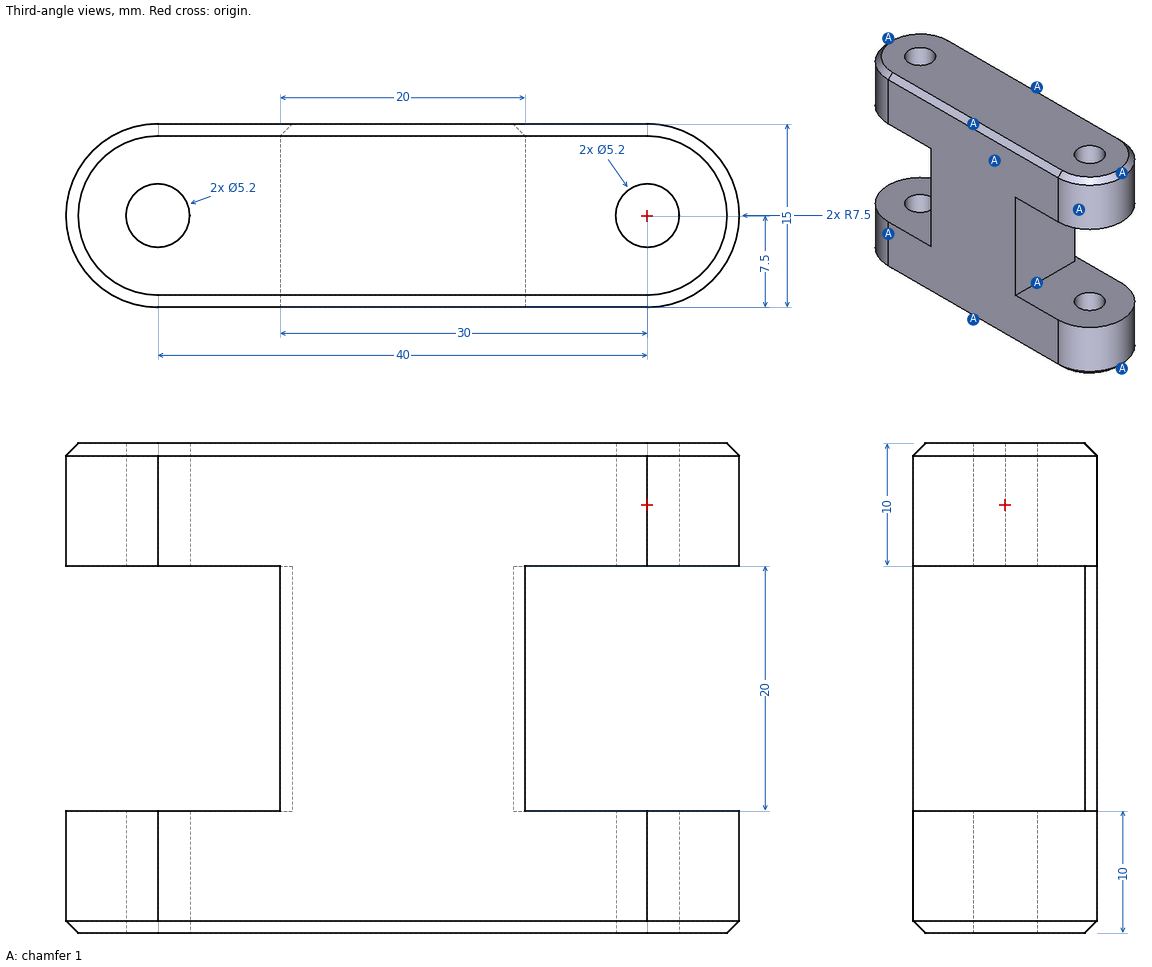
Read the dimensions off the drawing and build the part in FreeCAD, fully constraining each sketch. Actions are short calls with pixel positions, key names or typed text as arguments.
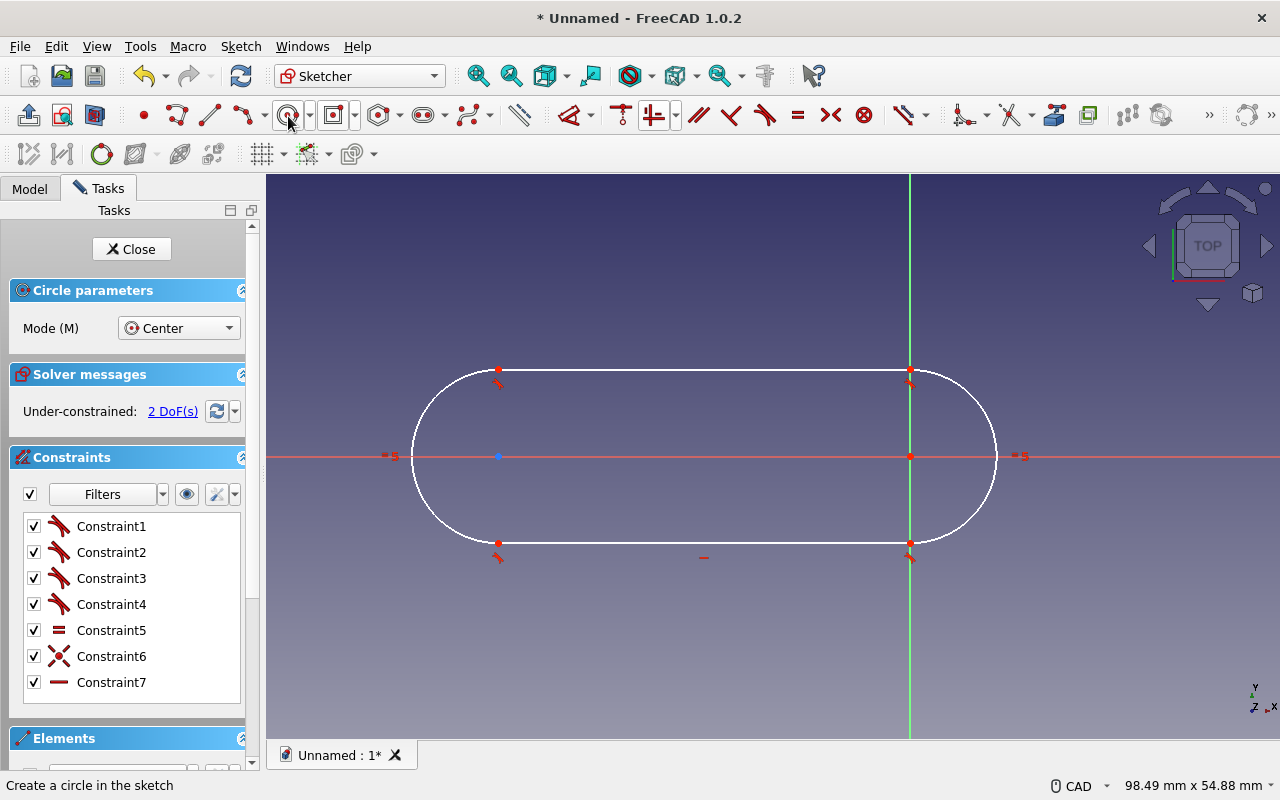
click(910, 456)
move(929, 438)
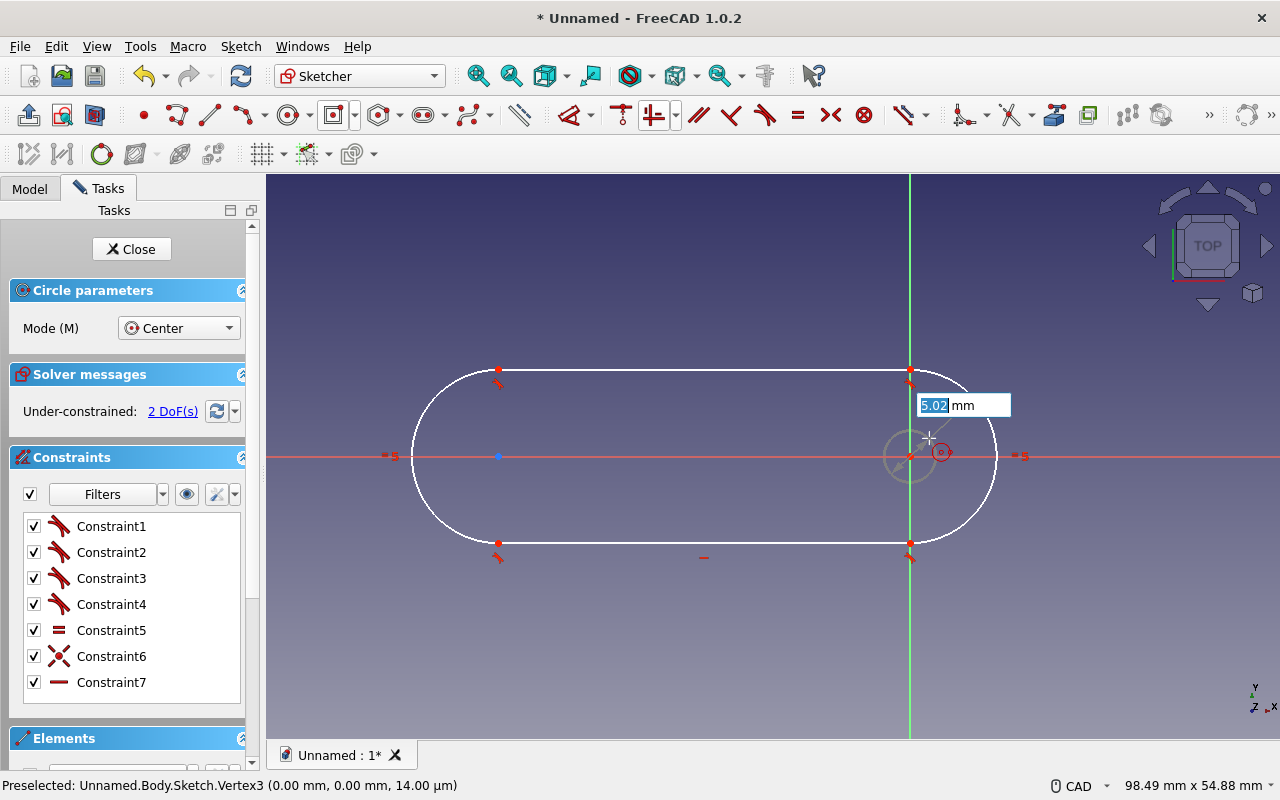
text(5.2)
key(Return)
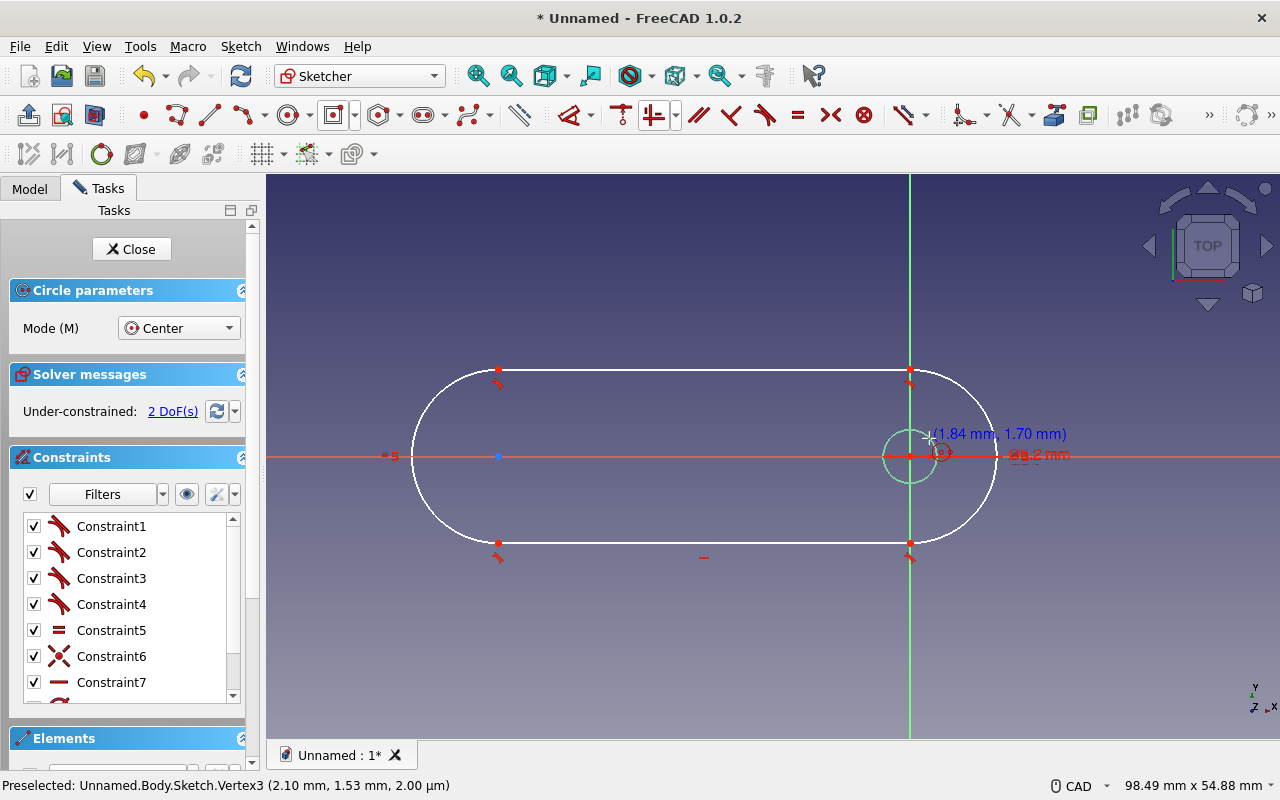
click(499, 456)
move(517, 438)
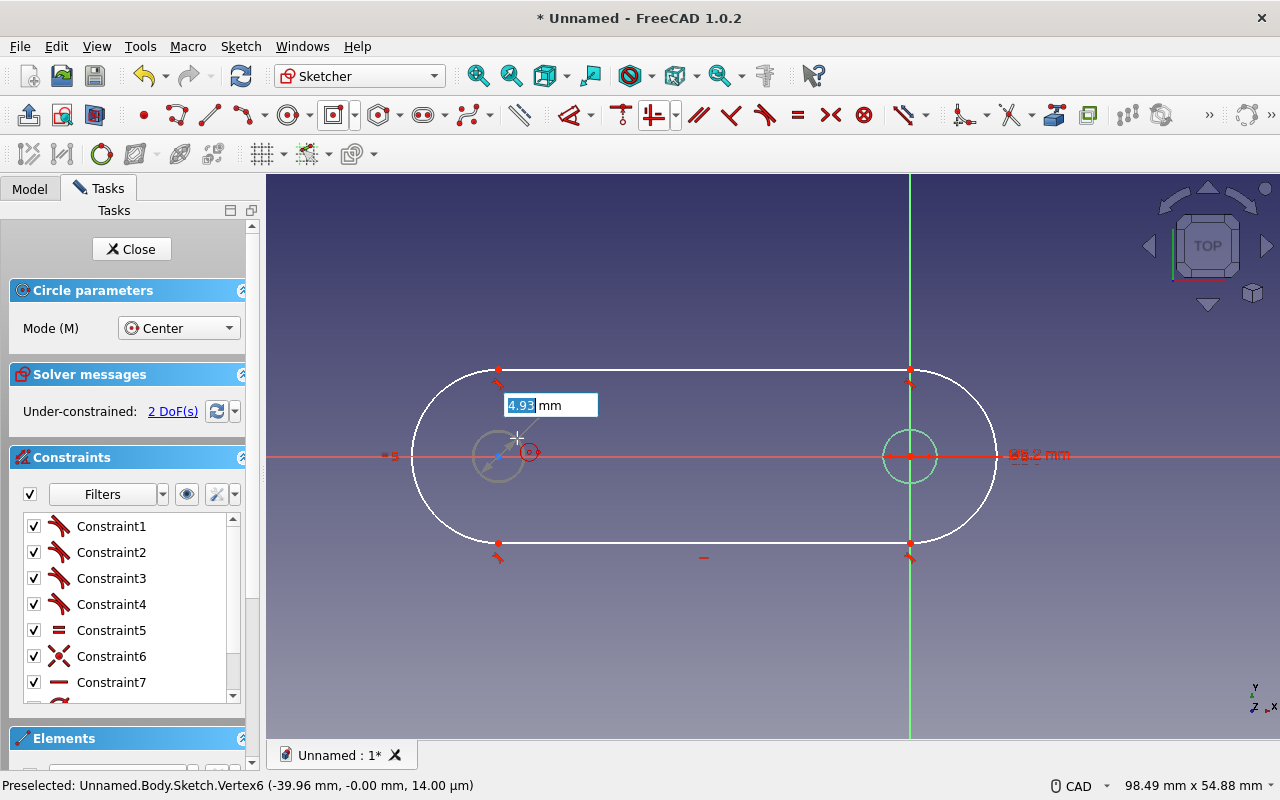
text(5.2)
key(Return)
key(Escape)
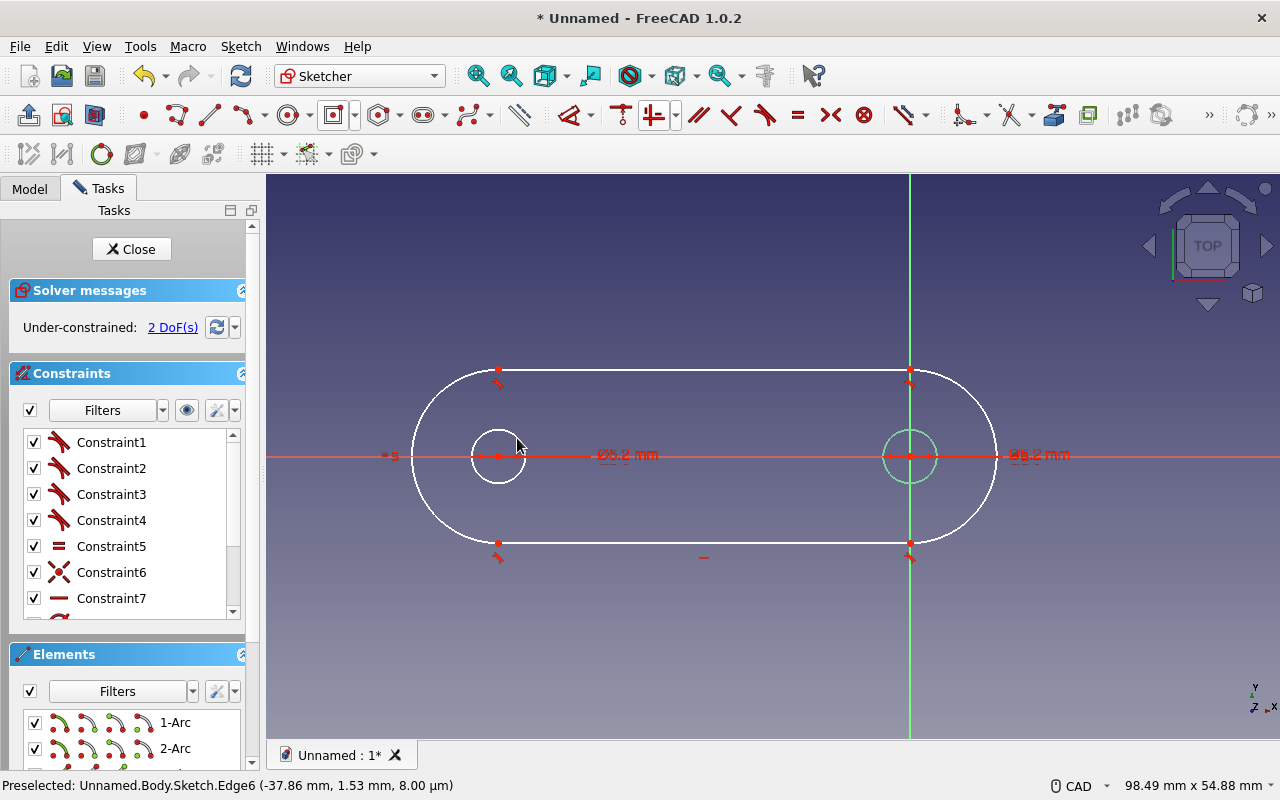
click(568, 116)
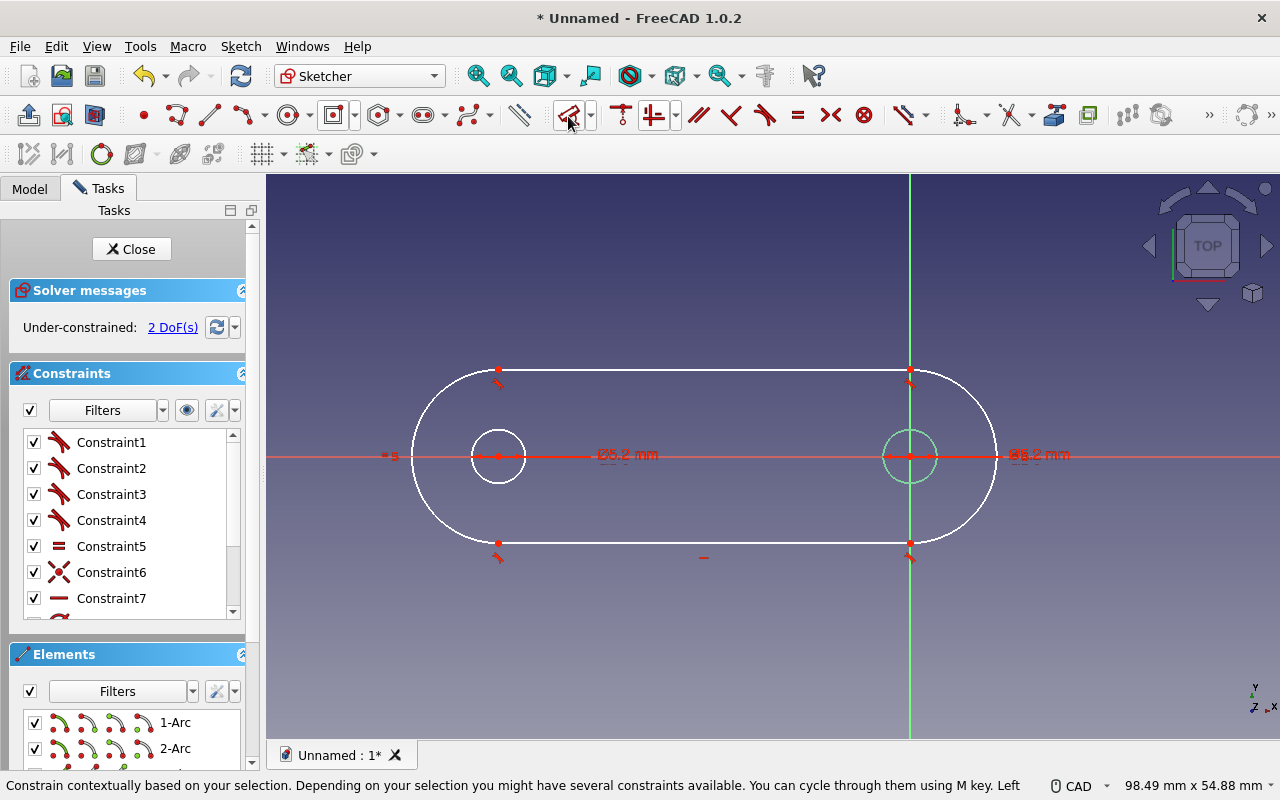
click(980, 507)
click(1006, 526)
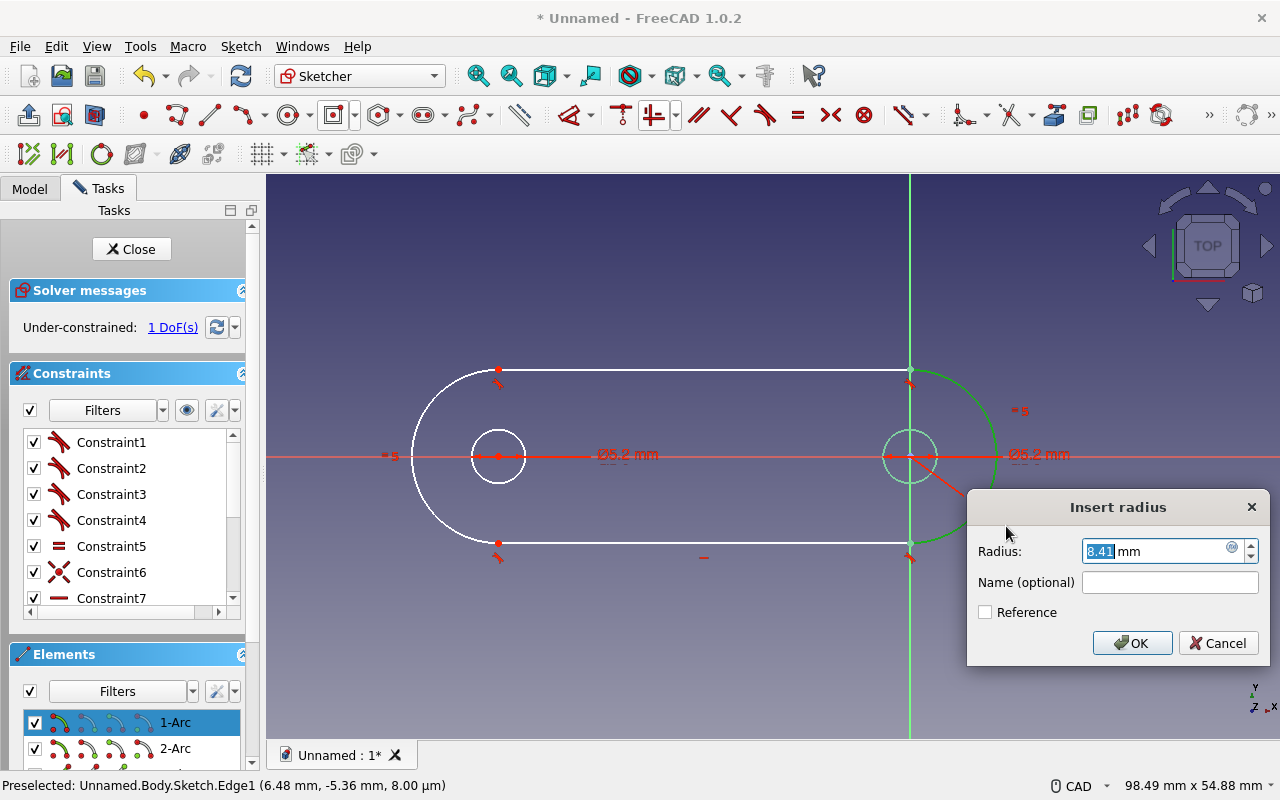
text(7.5)
key(Return)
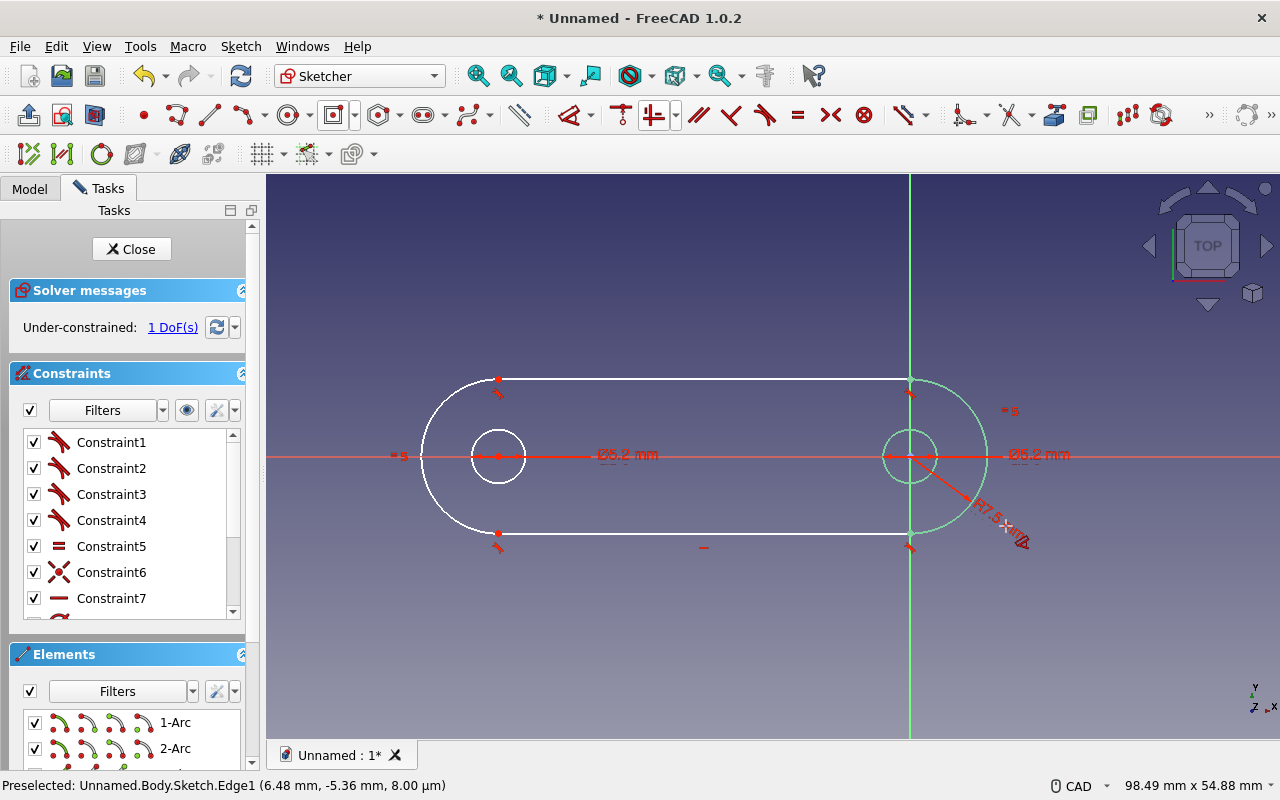
click(787, 534)
click(704, 568)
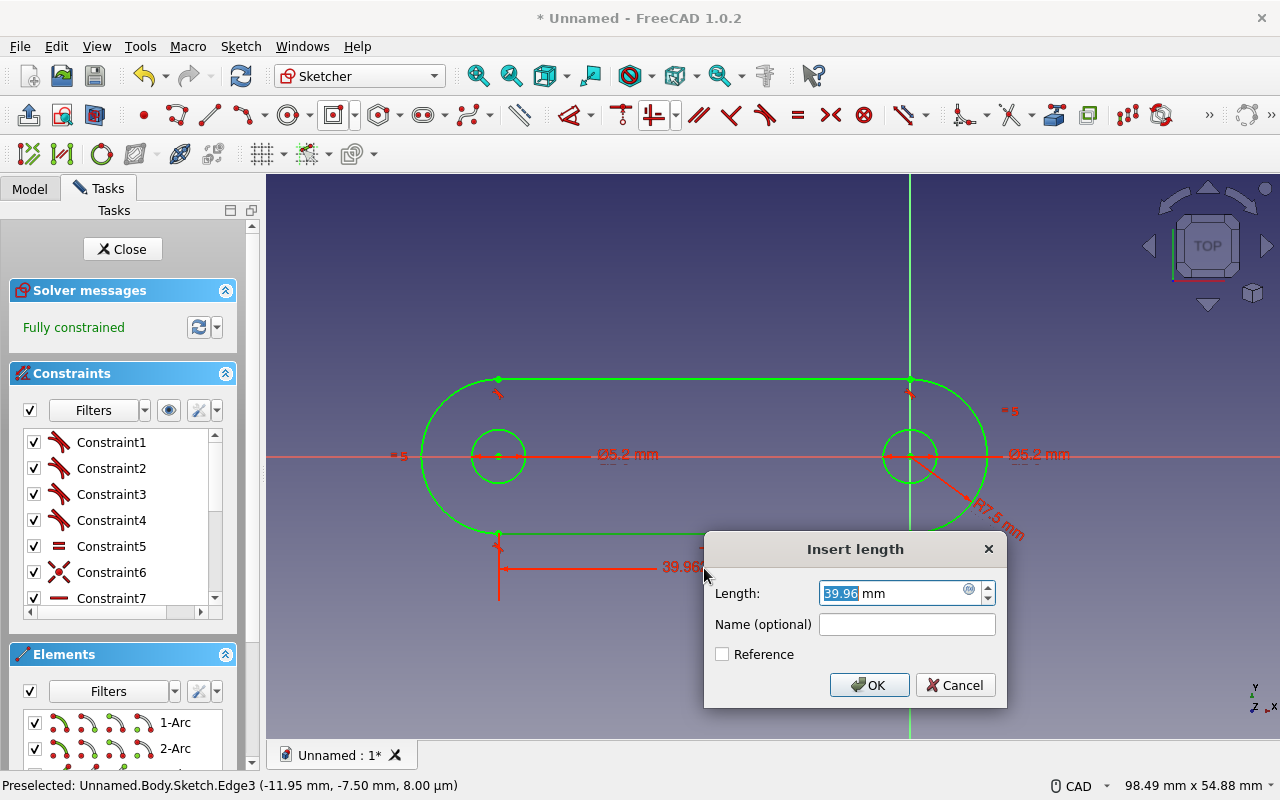
text(40)
key(Return)
key(Escape)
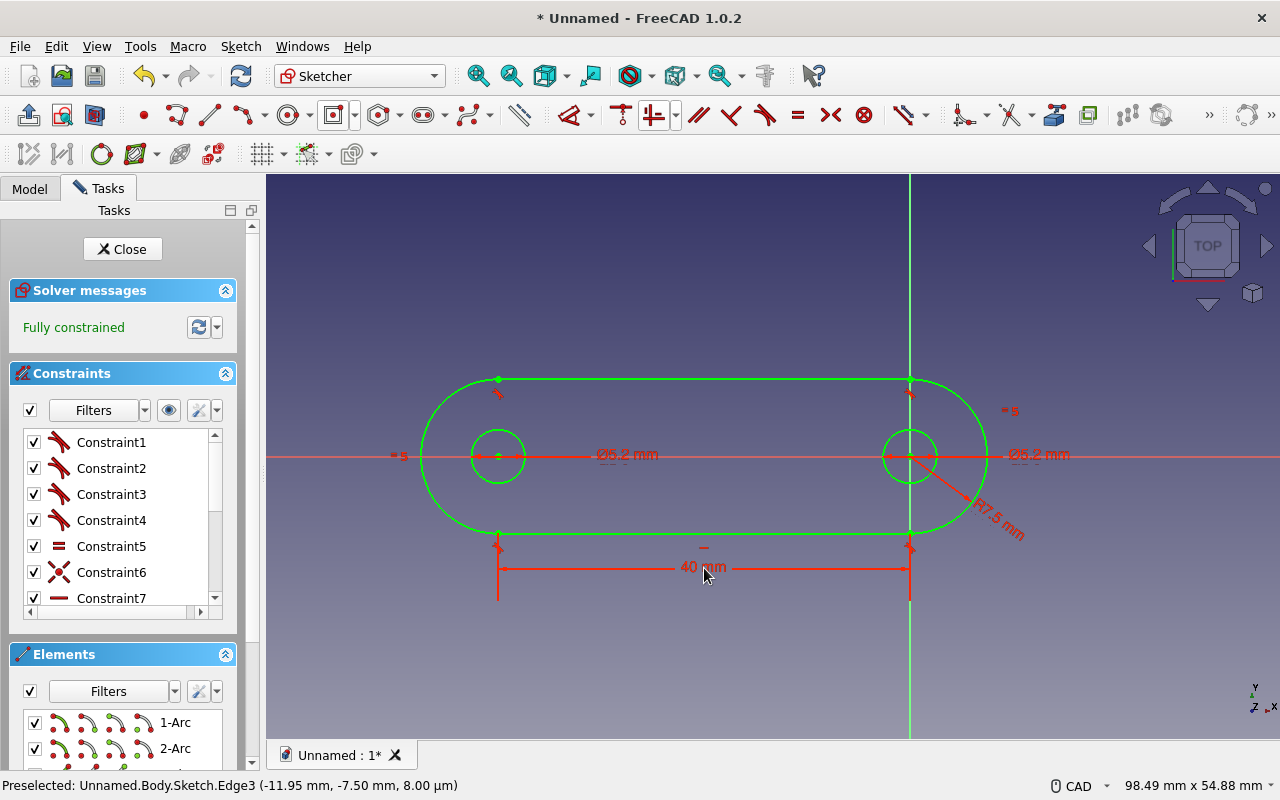
click(123, 249)